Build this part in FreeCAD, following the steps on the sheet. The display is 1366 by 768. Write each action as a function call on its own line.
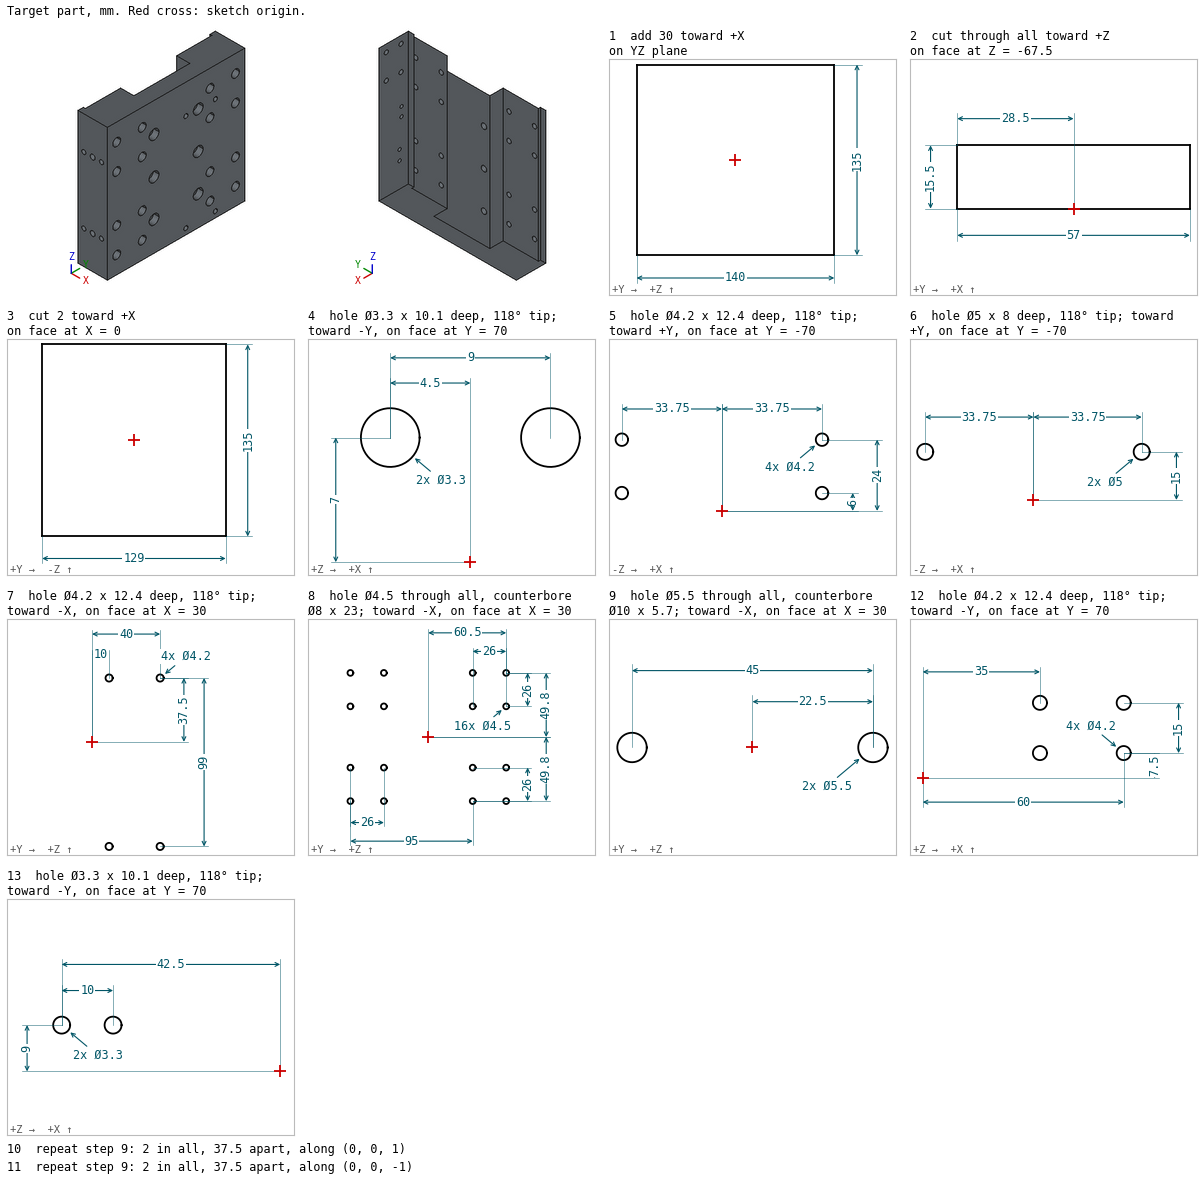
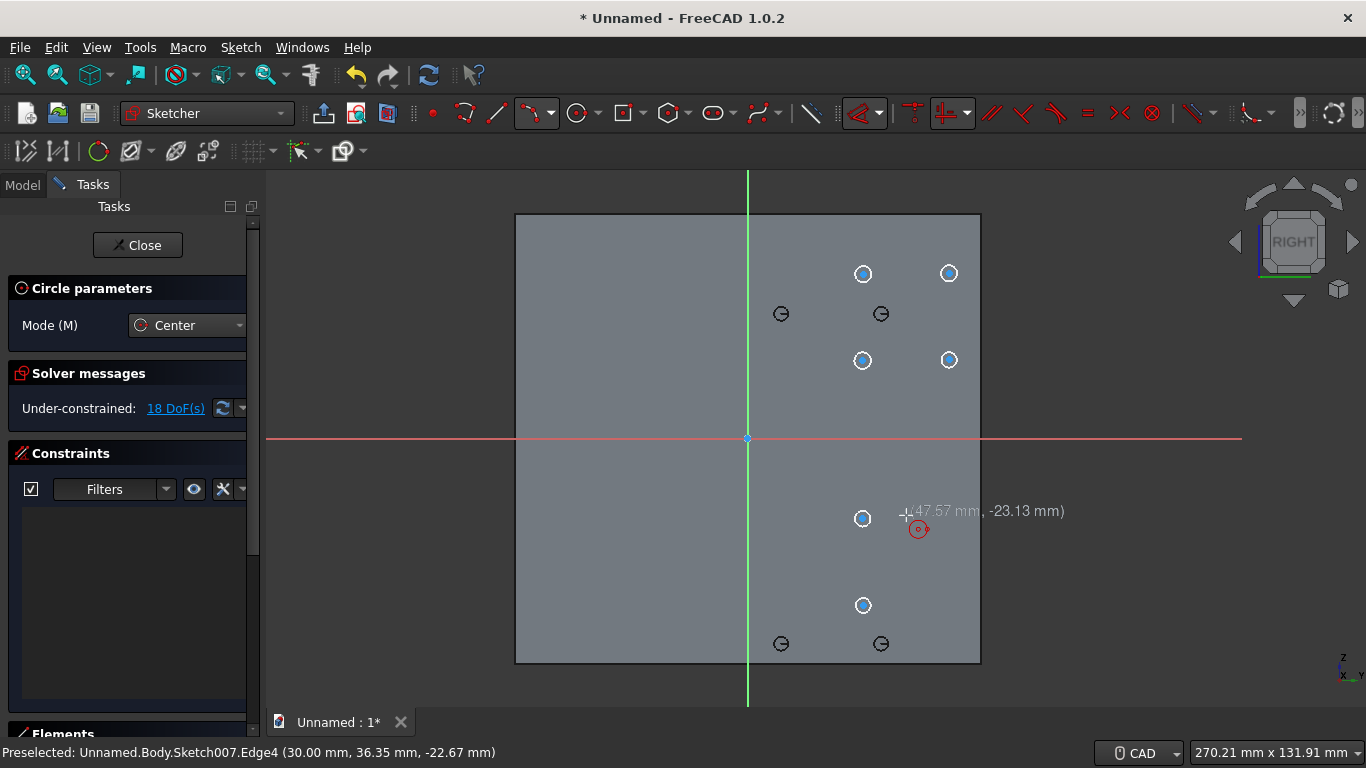
click(950, 518)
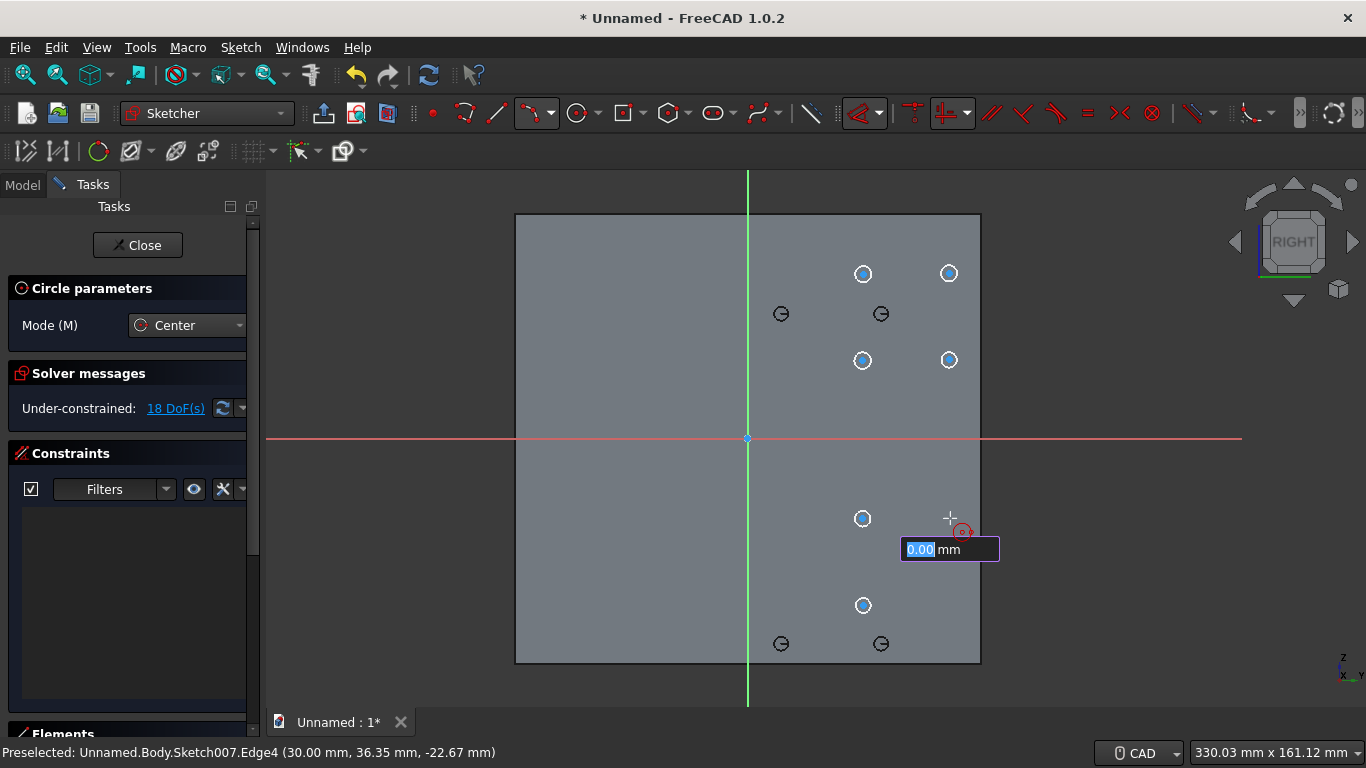
scroll(955, 513, up, 4)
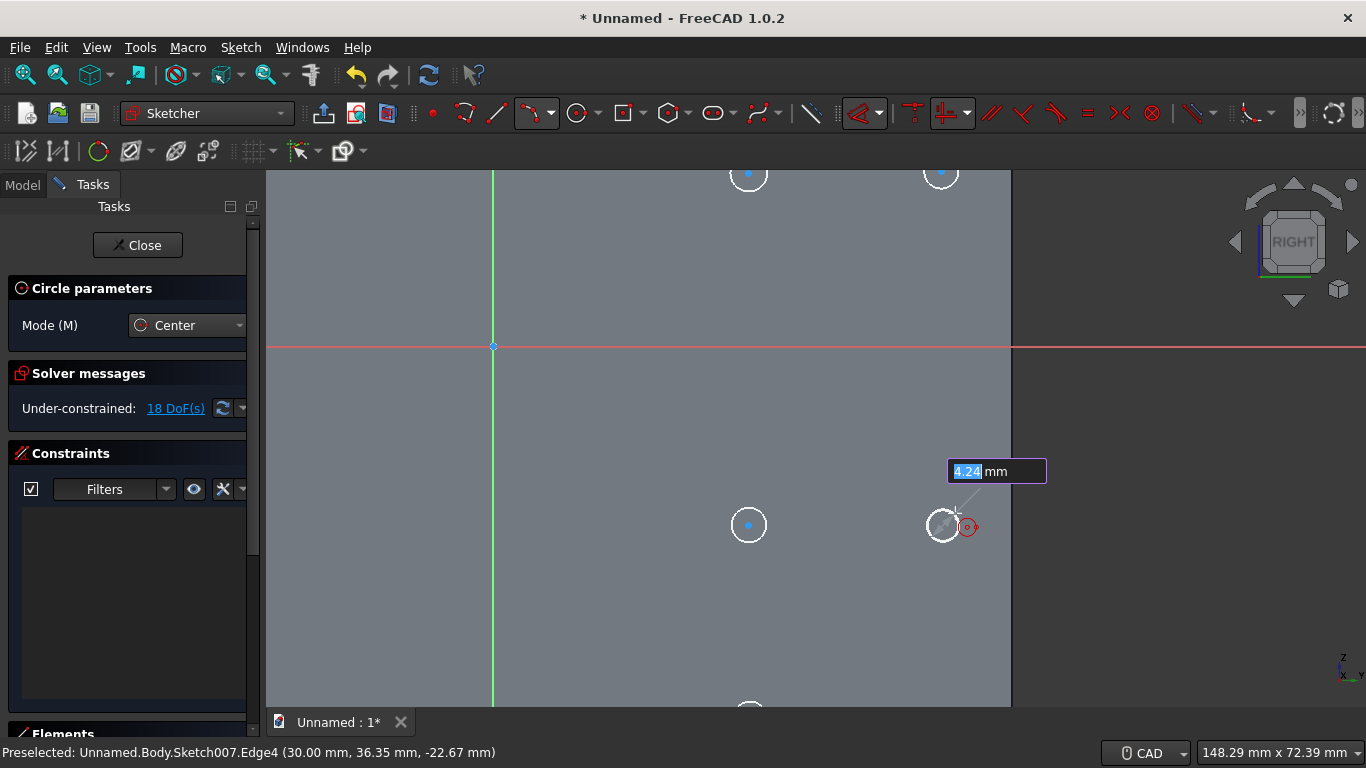
click(954, 512)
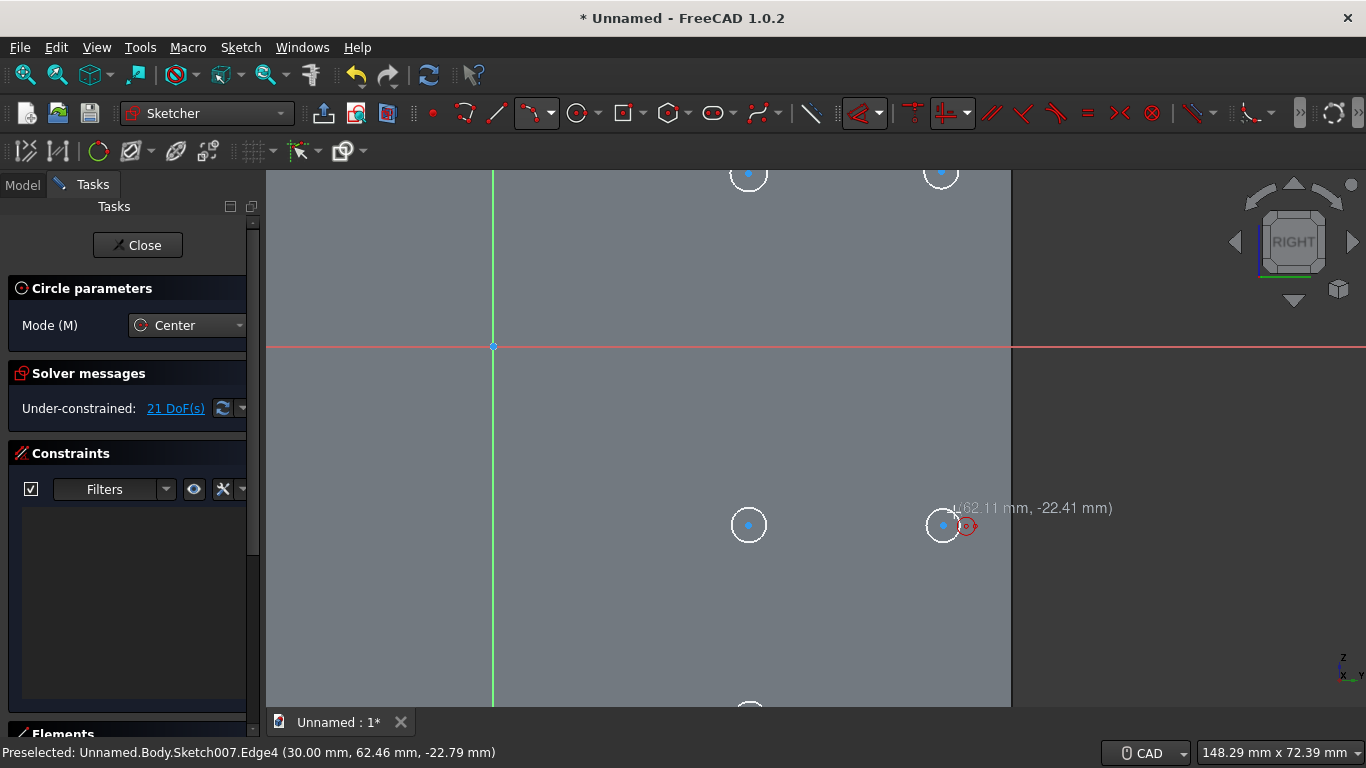
scroll(955, 513, down, 4)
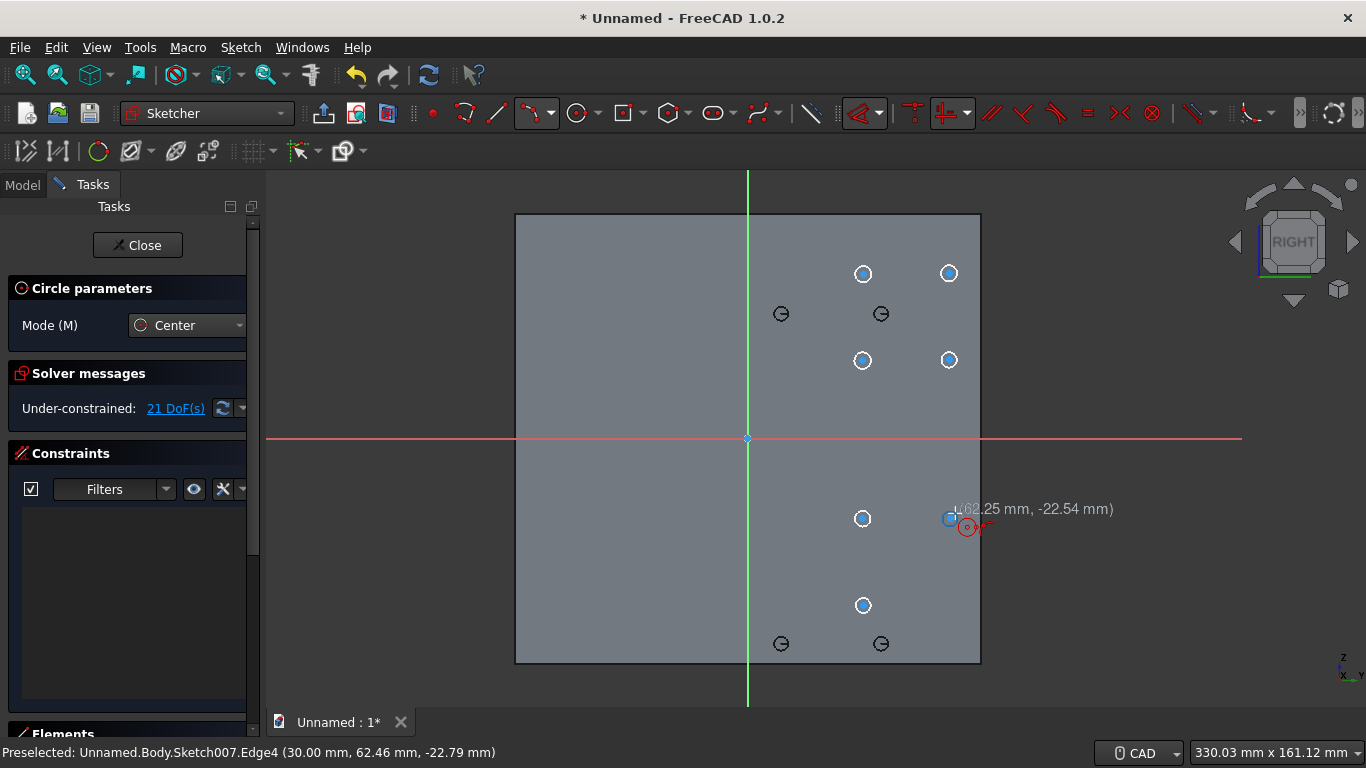
scroll(950, 605, up, 6)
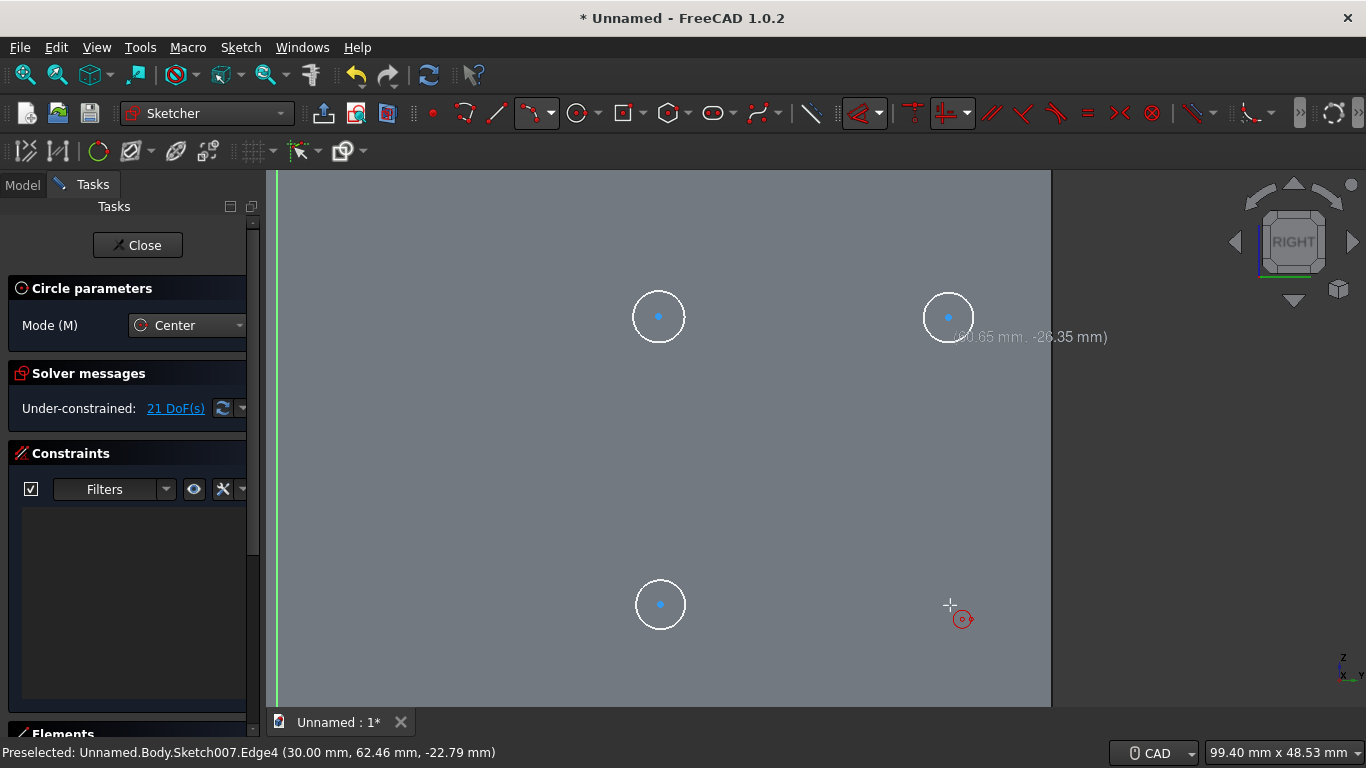
scroll(950, 606, down, 6)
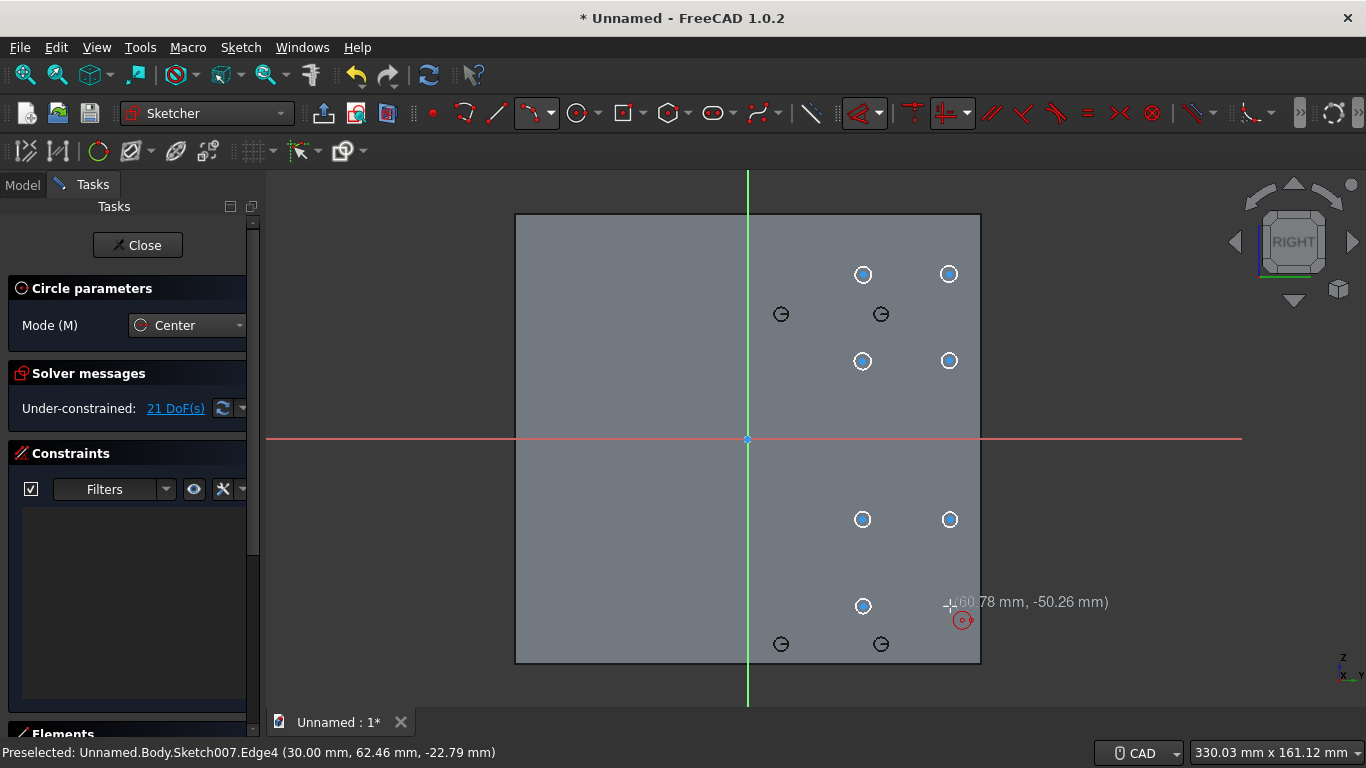
click(950, 605)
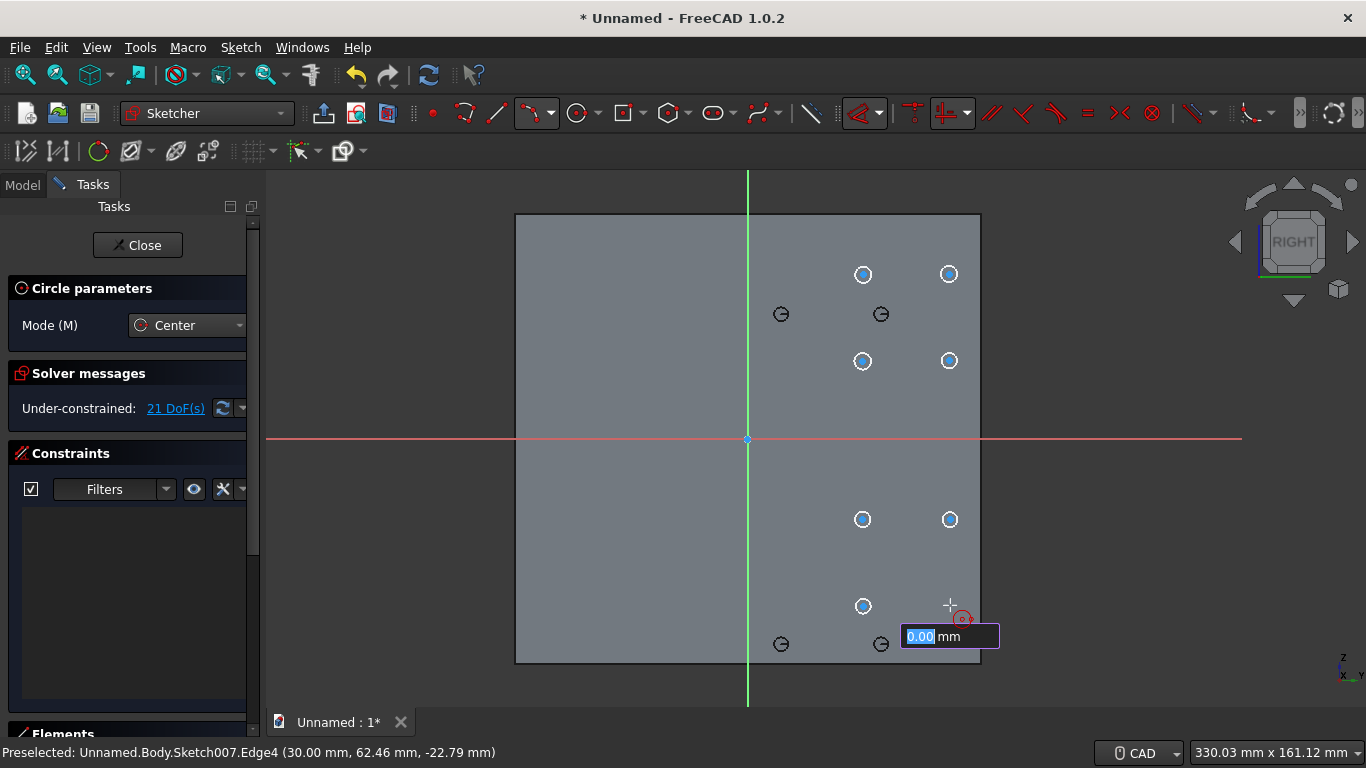
scroll(955, 600, up, 4)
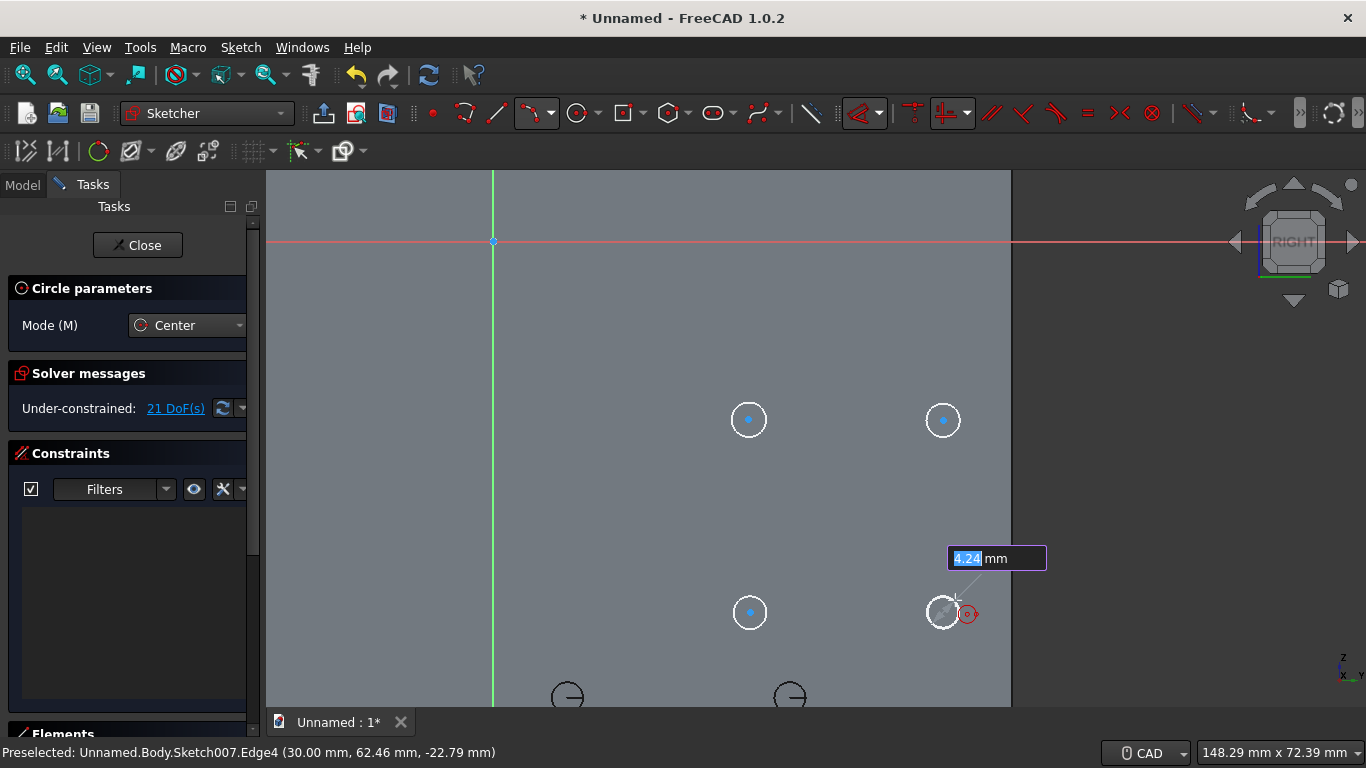
click(954, 599)